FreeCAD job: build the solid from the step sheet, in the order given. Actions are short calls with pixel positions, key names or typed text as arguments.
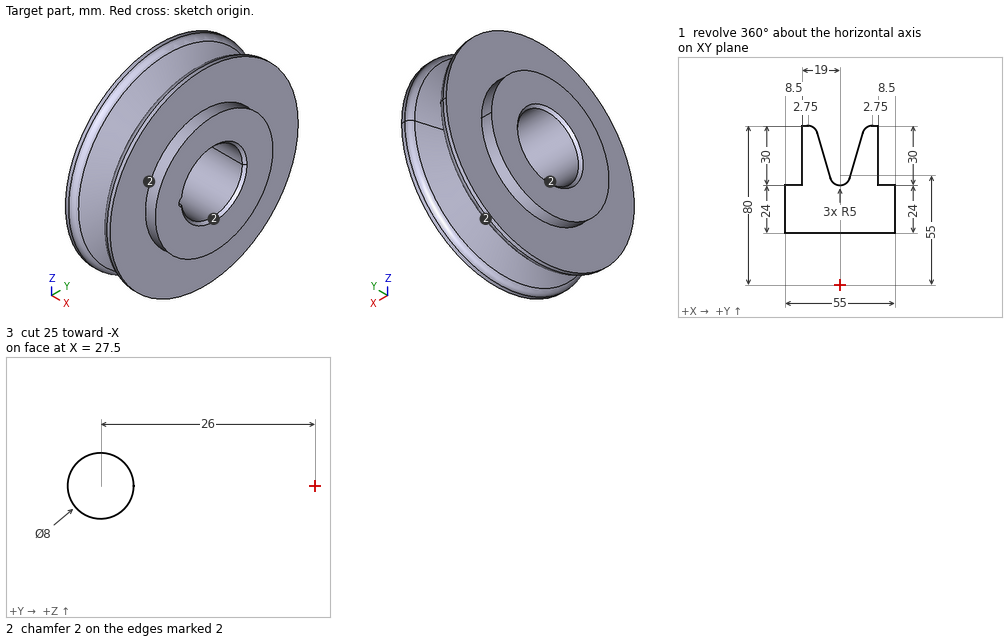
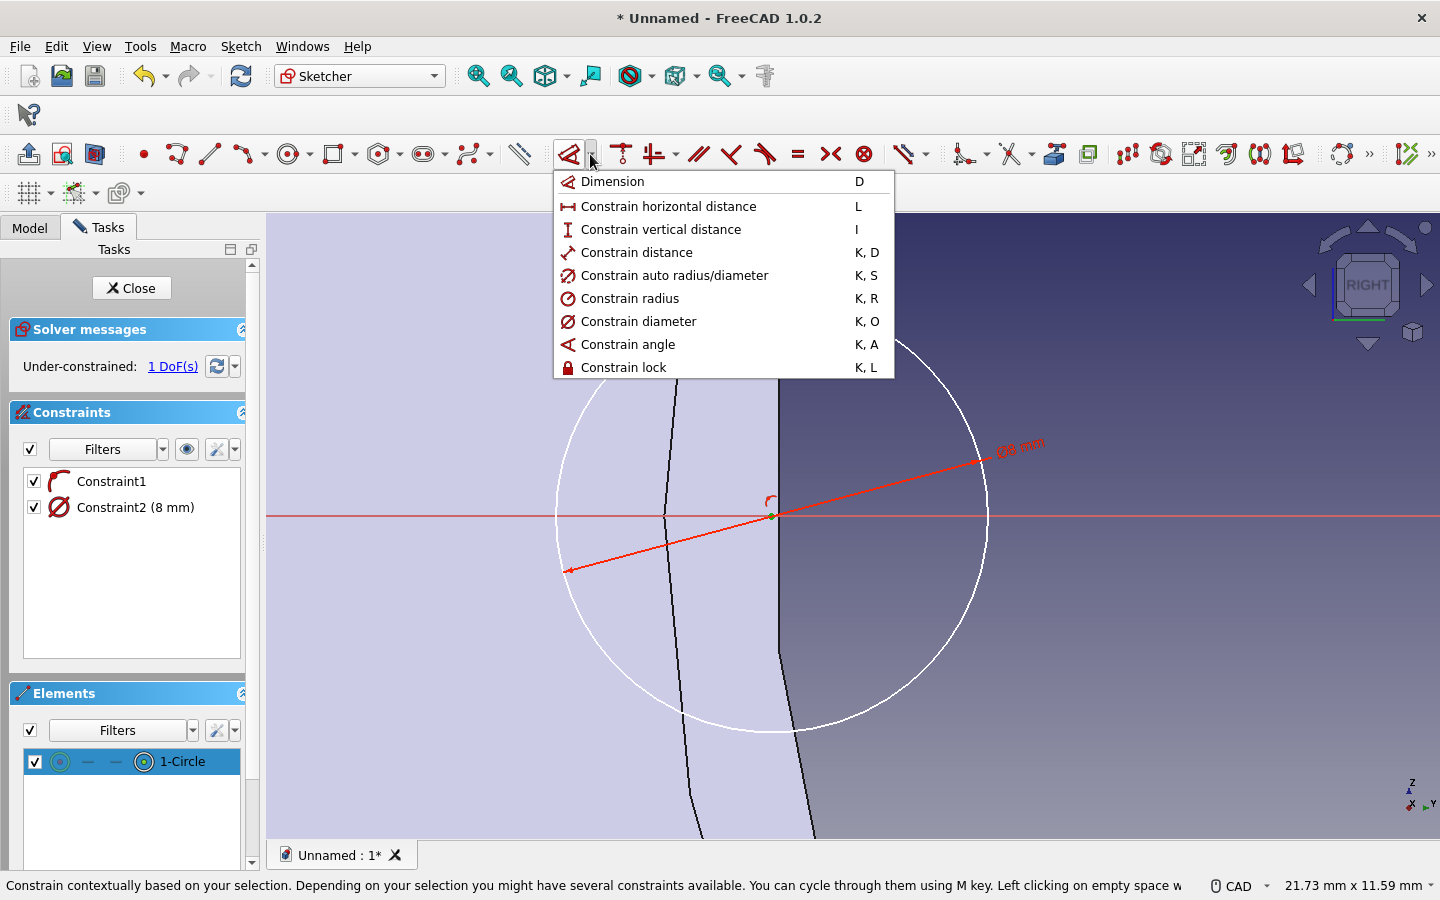
click(724, 206)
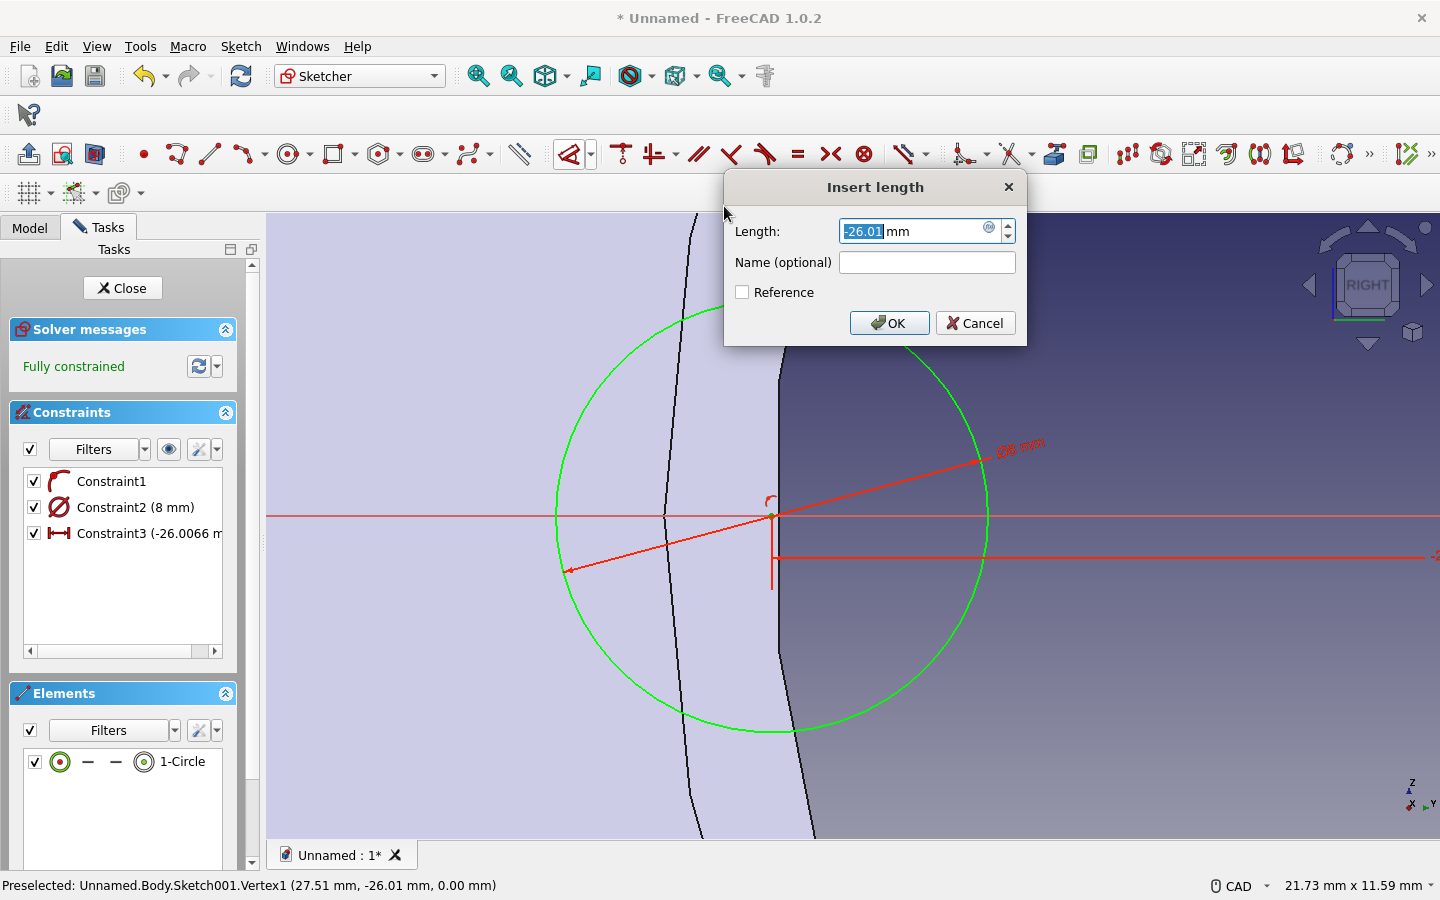
text(-26)
key(Return)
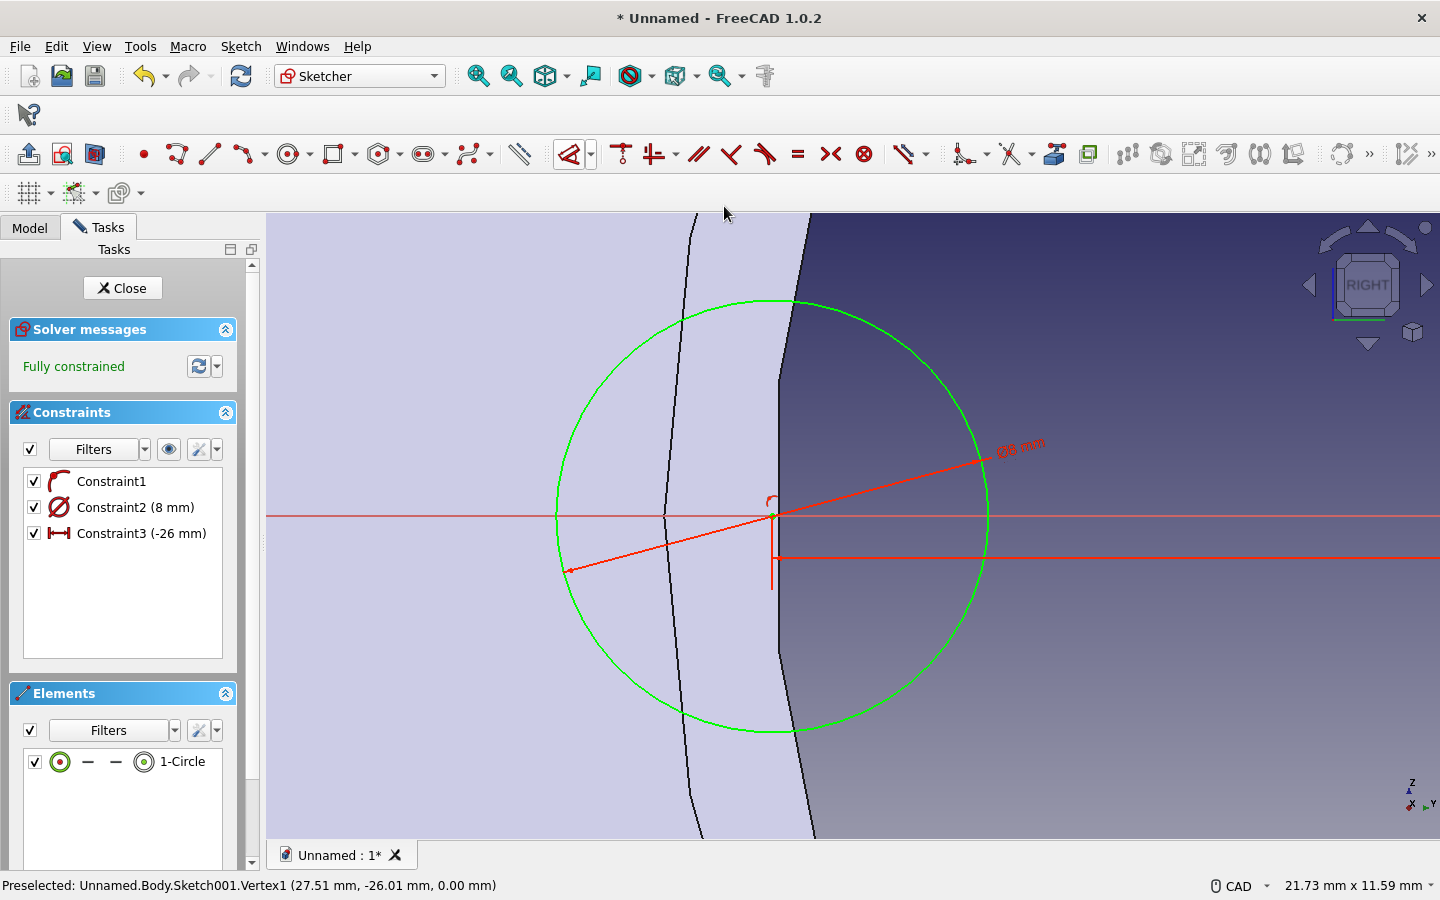
click(123, 288)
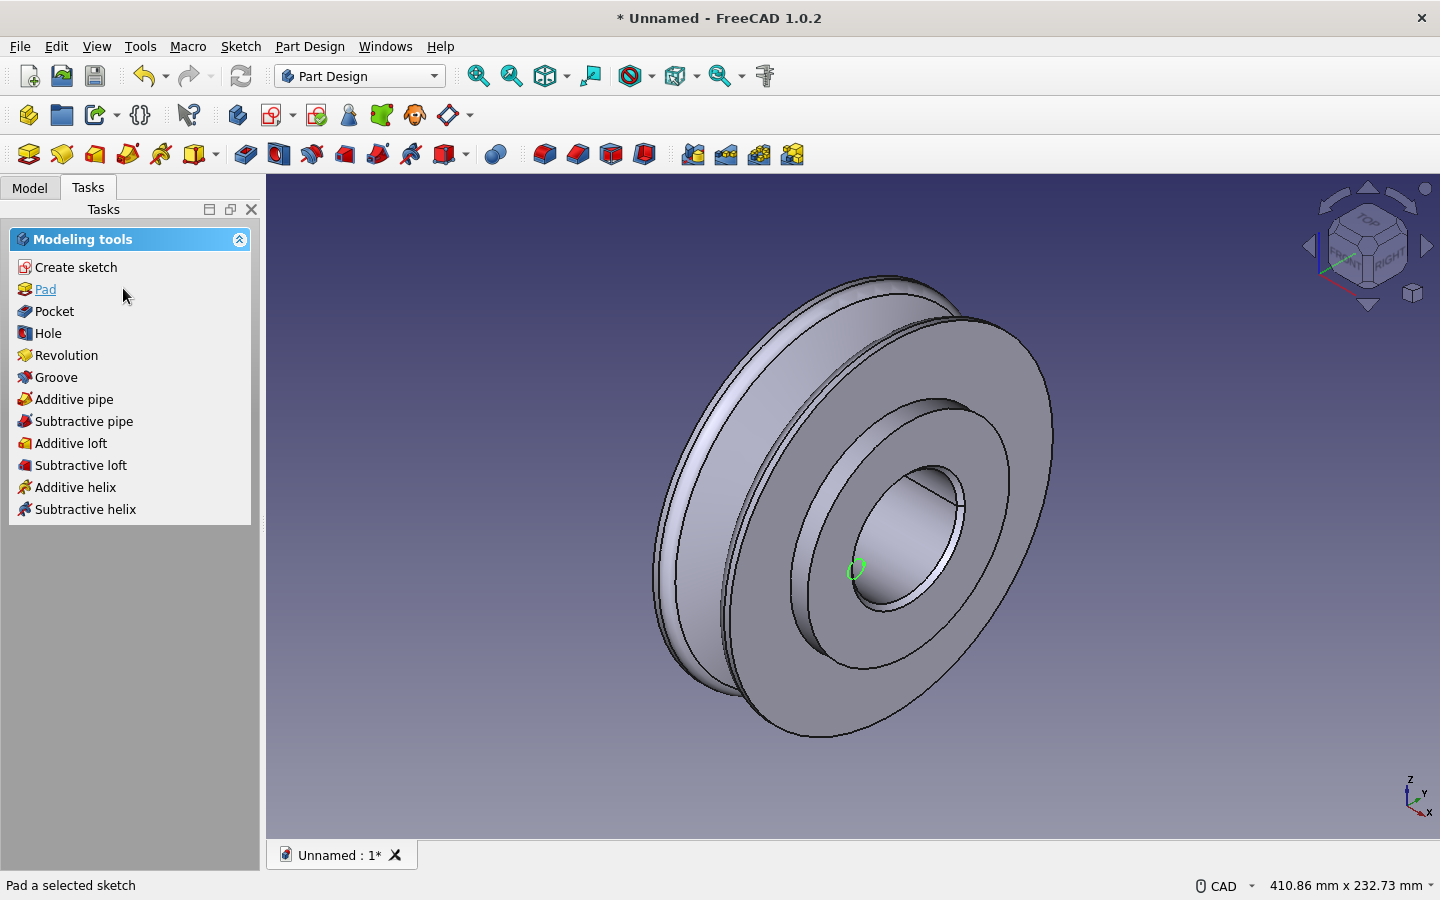
click(246, 154)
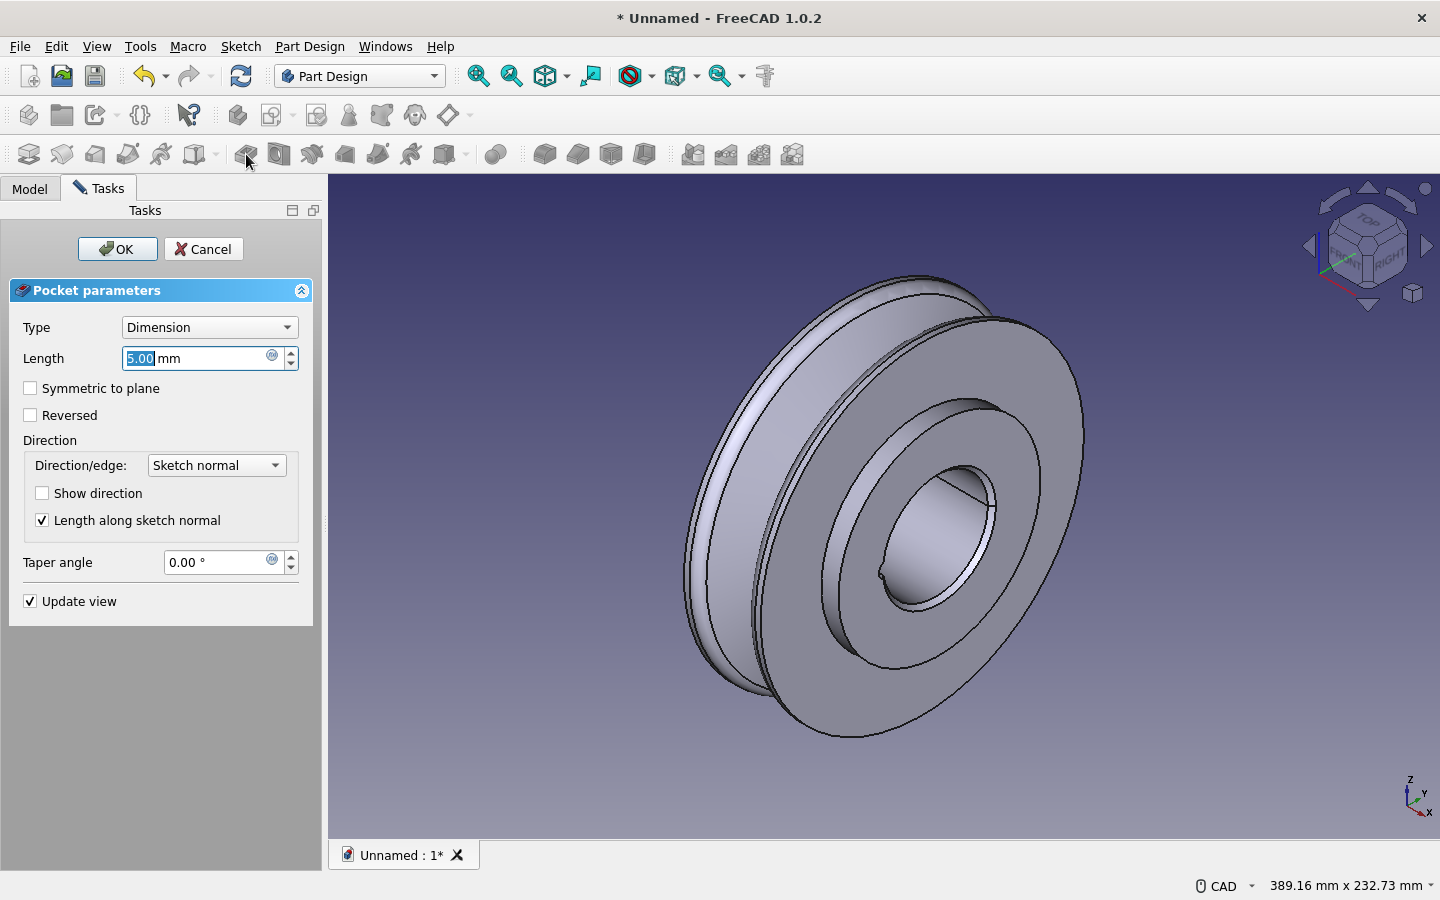
text(25)
key(Tab)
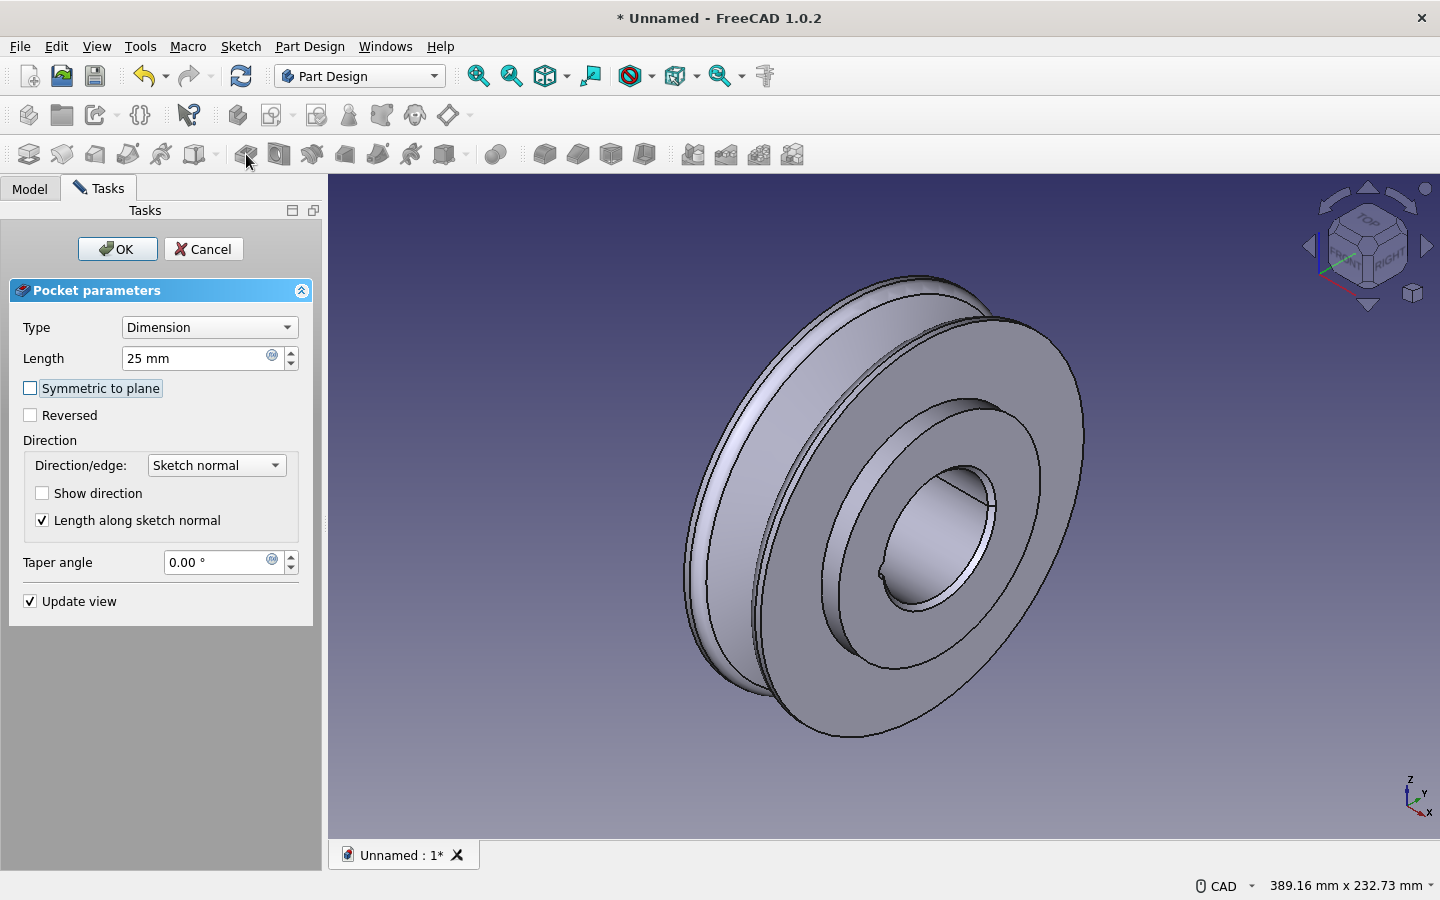
click(118, 249)